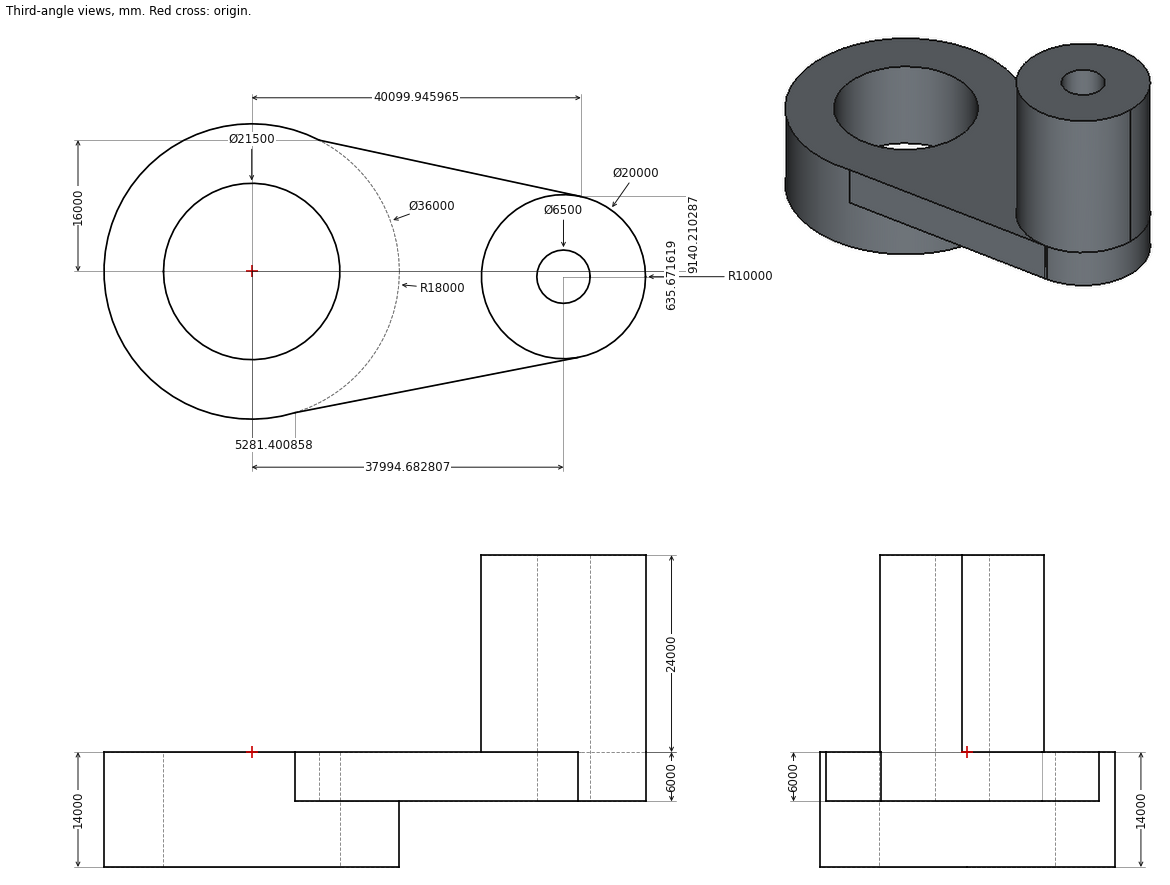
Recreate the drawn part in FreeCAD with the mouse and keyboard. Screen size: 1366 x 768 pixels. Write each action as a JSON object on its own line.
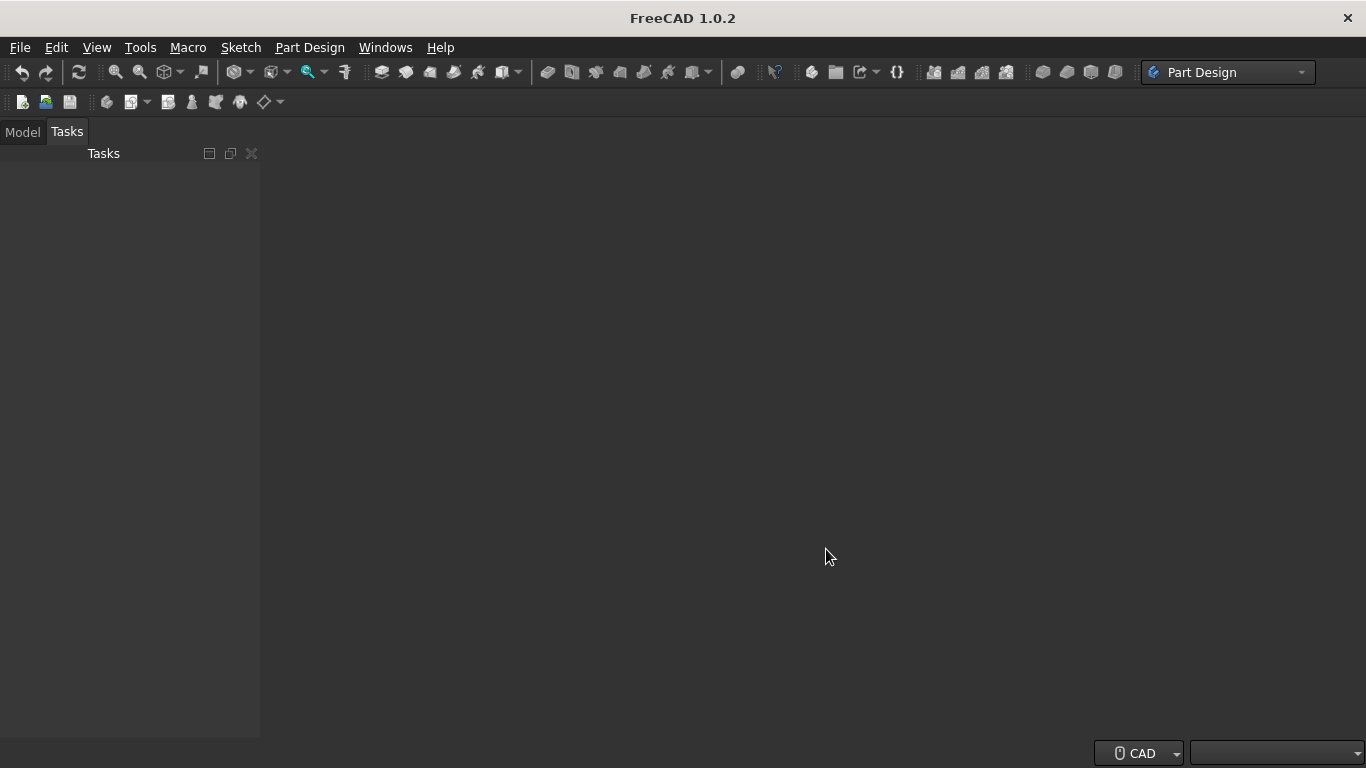
{"action": "left_click", "coordinate": [22, 102]}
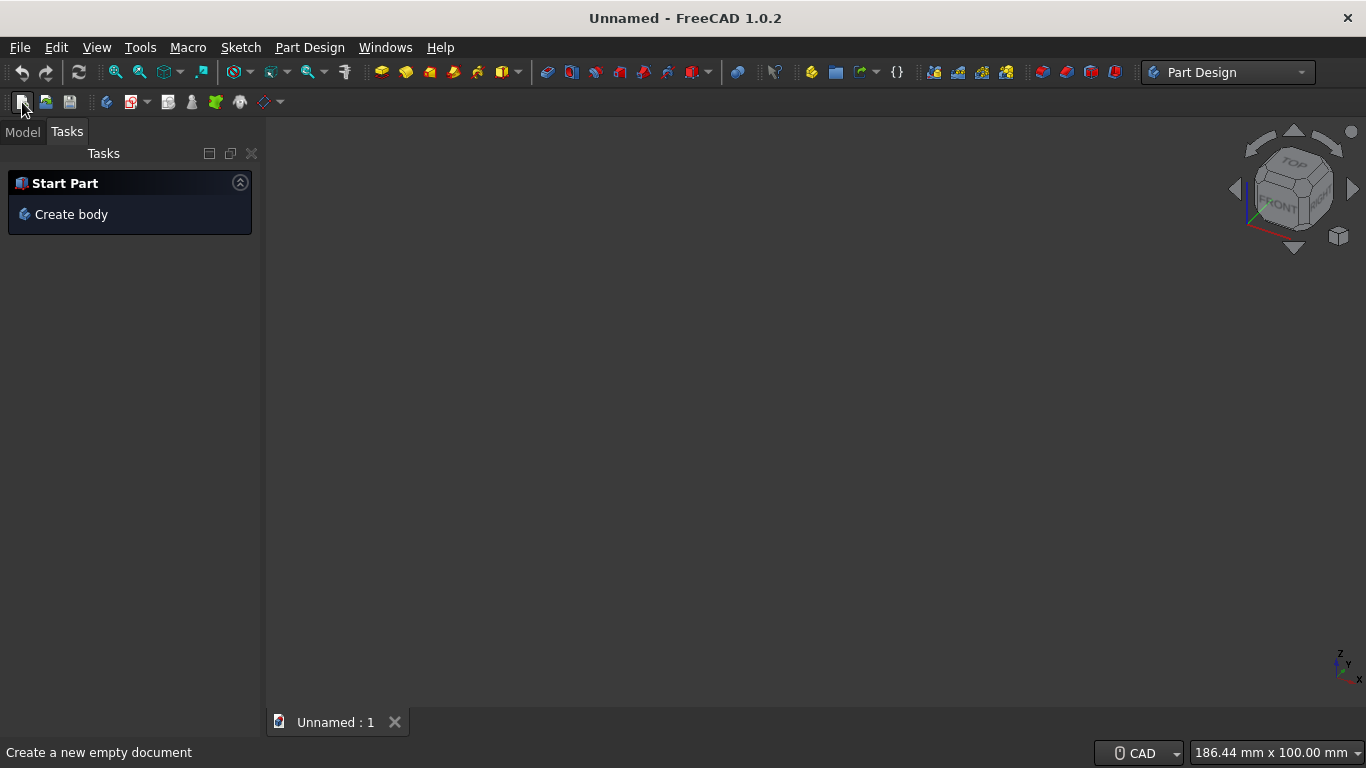
{"action": "left_click", "coordinate": [132, 102]}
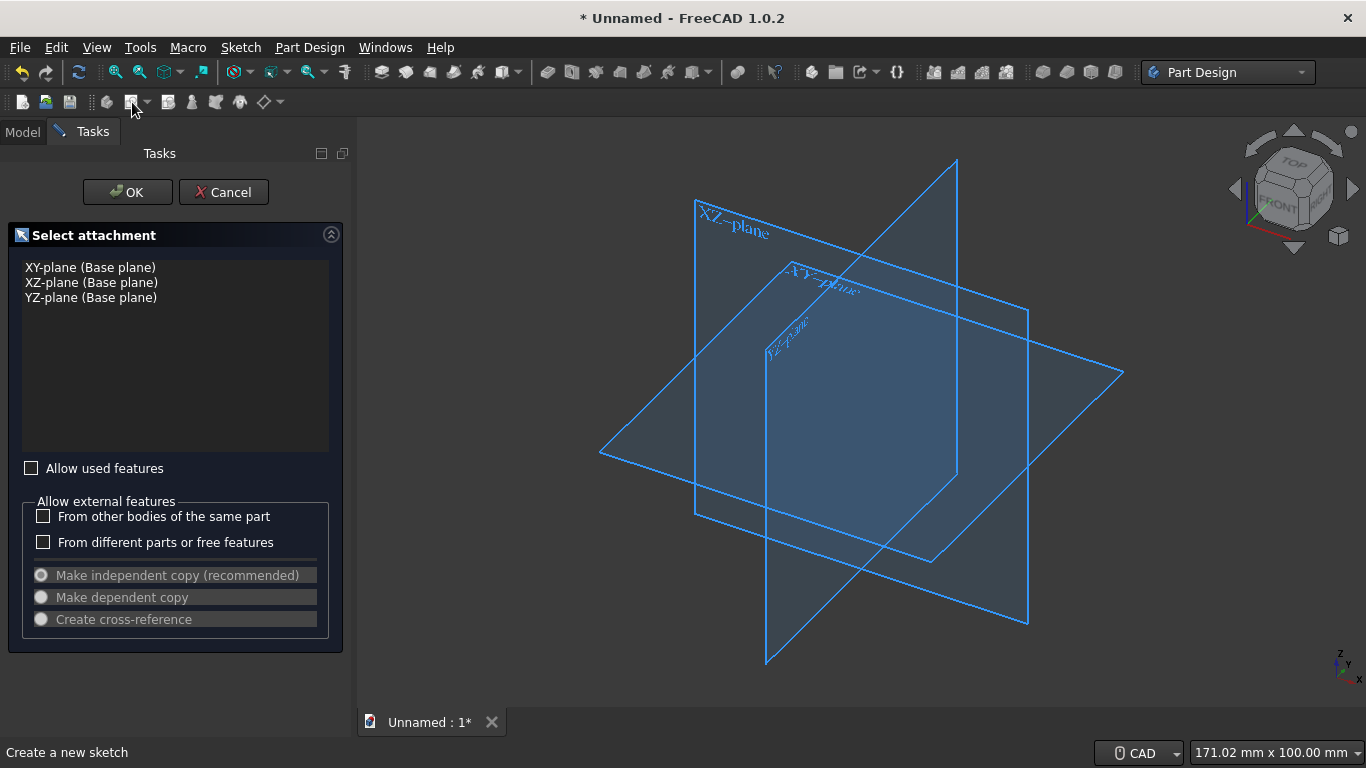
{"action": "left_click", "coordinate": [82, 268]}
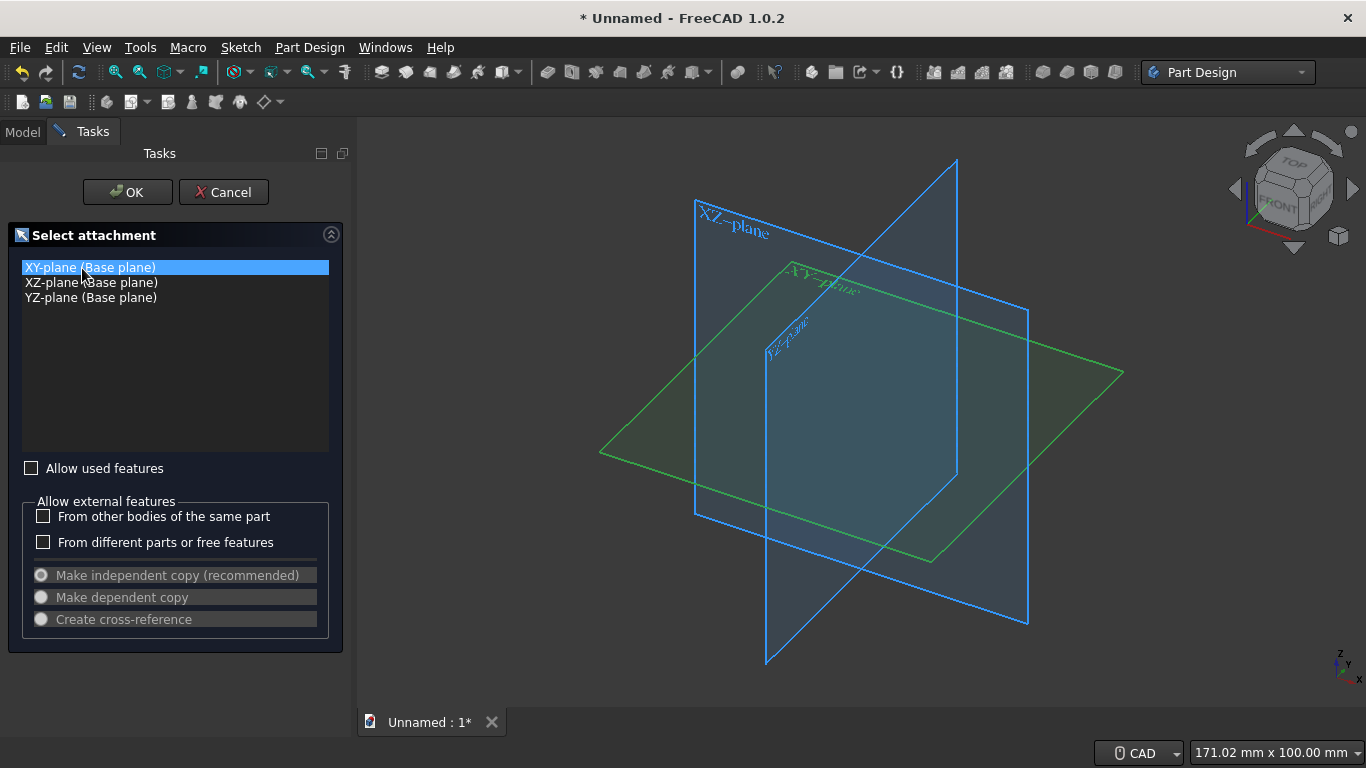
{"action": "left_click", "coordinate": [128, 192]}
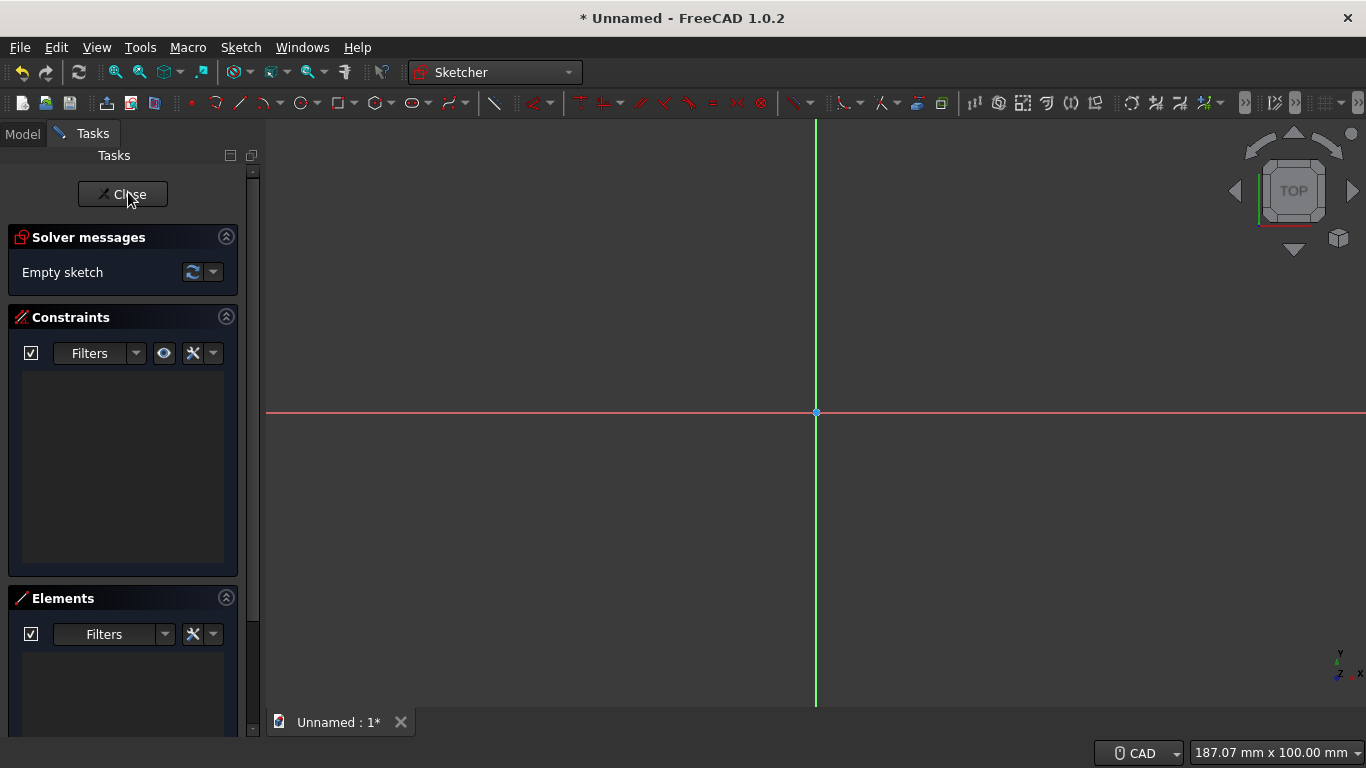
{"action": "scroll", "coordinate": [748, 413], "scroll_direction": "down", "scroll_amount": 15}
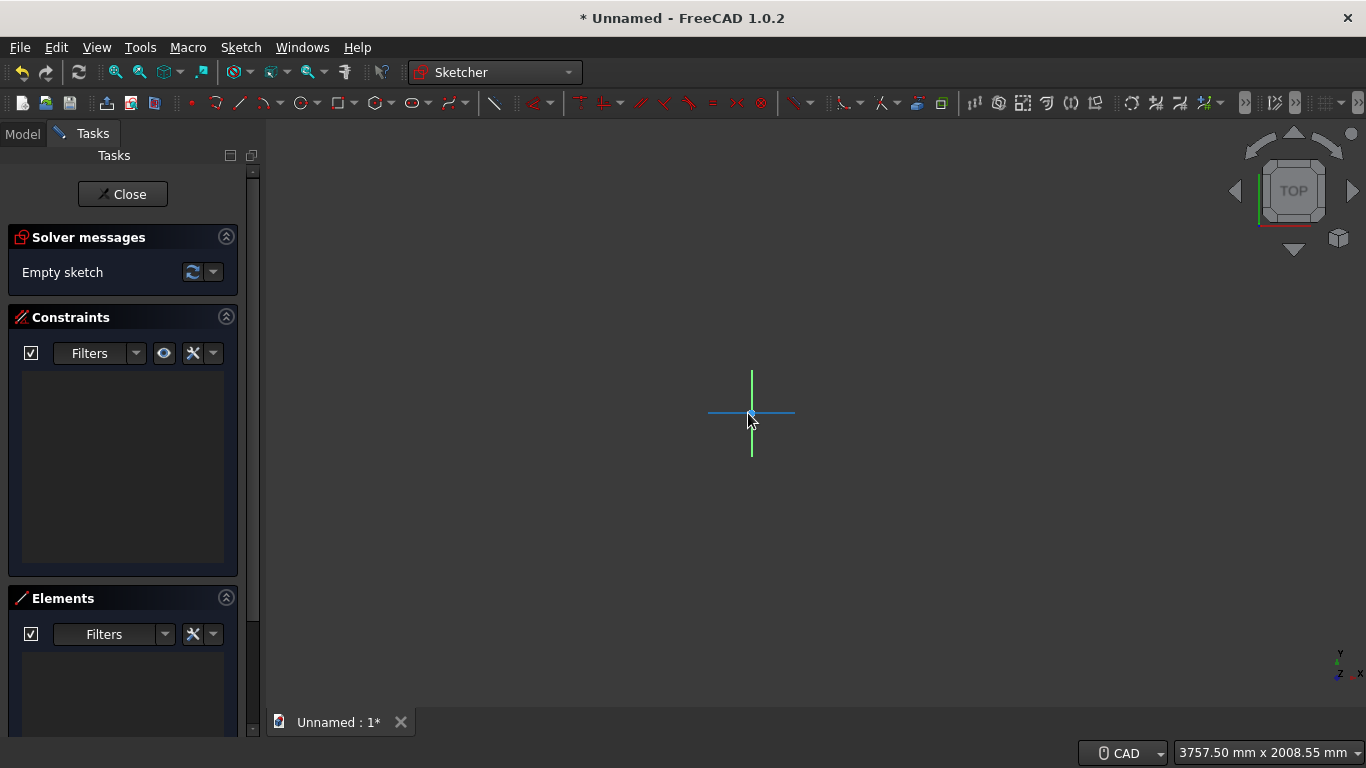
{"action": "scroll", "coordinate": [747, 413], "scroll_direction": "down", "scroll_amount": 16}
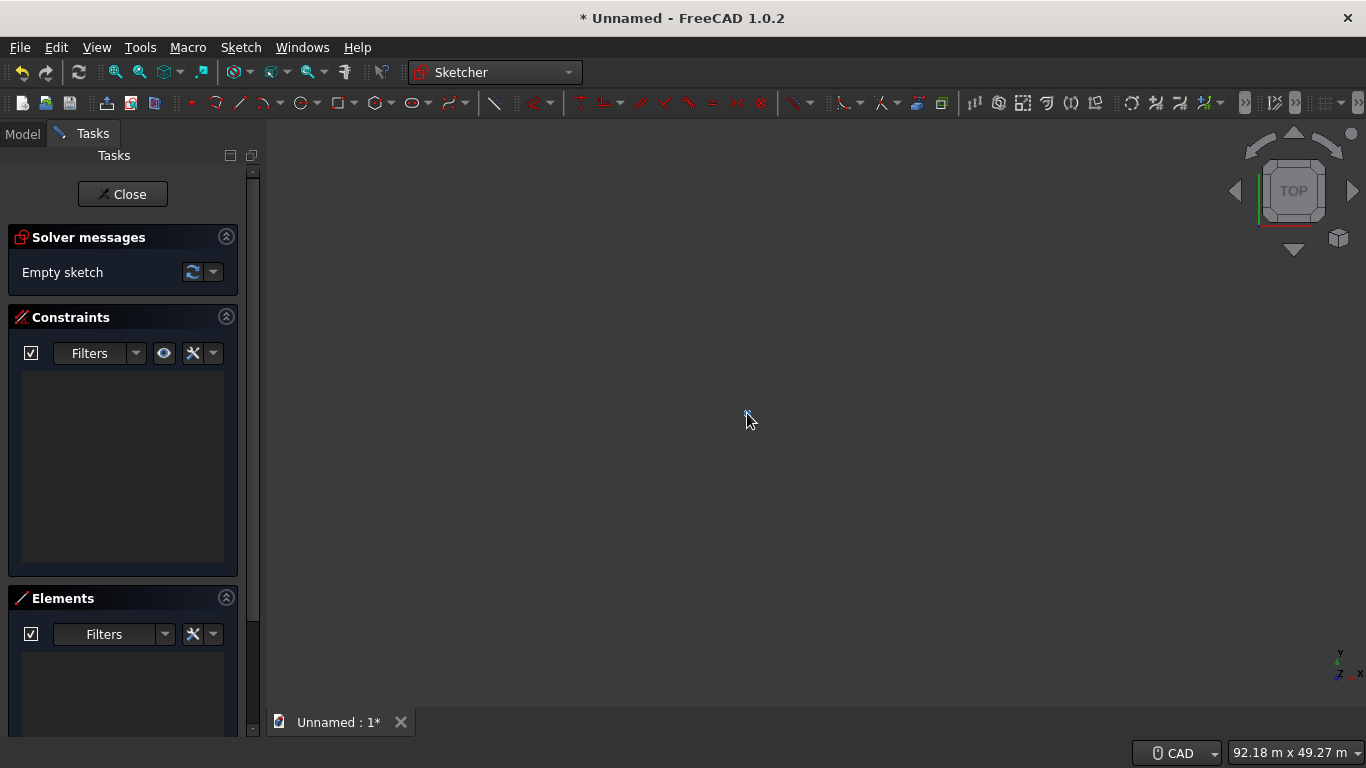
{"action": "left_click", "coordinate": [302, 104]}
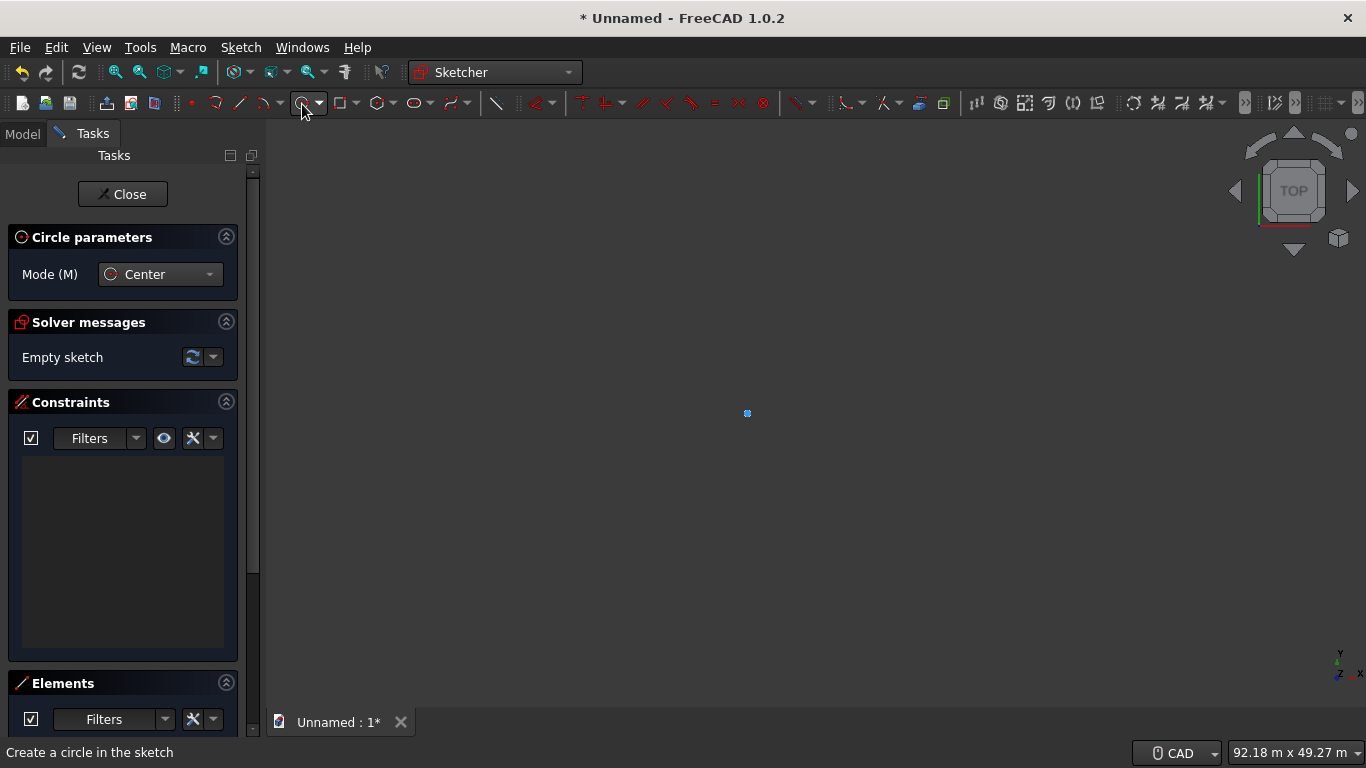
{"action": "left_click", "coordinate": [748, 413]}
{"action": "left_click", "coordinate": [899, 262]}
{"action": "key", "text": "Escape"}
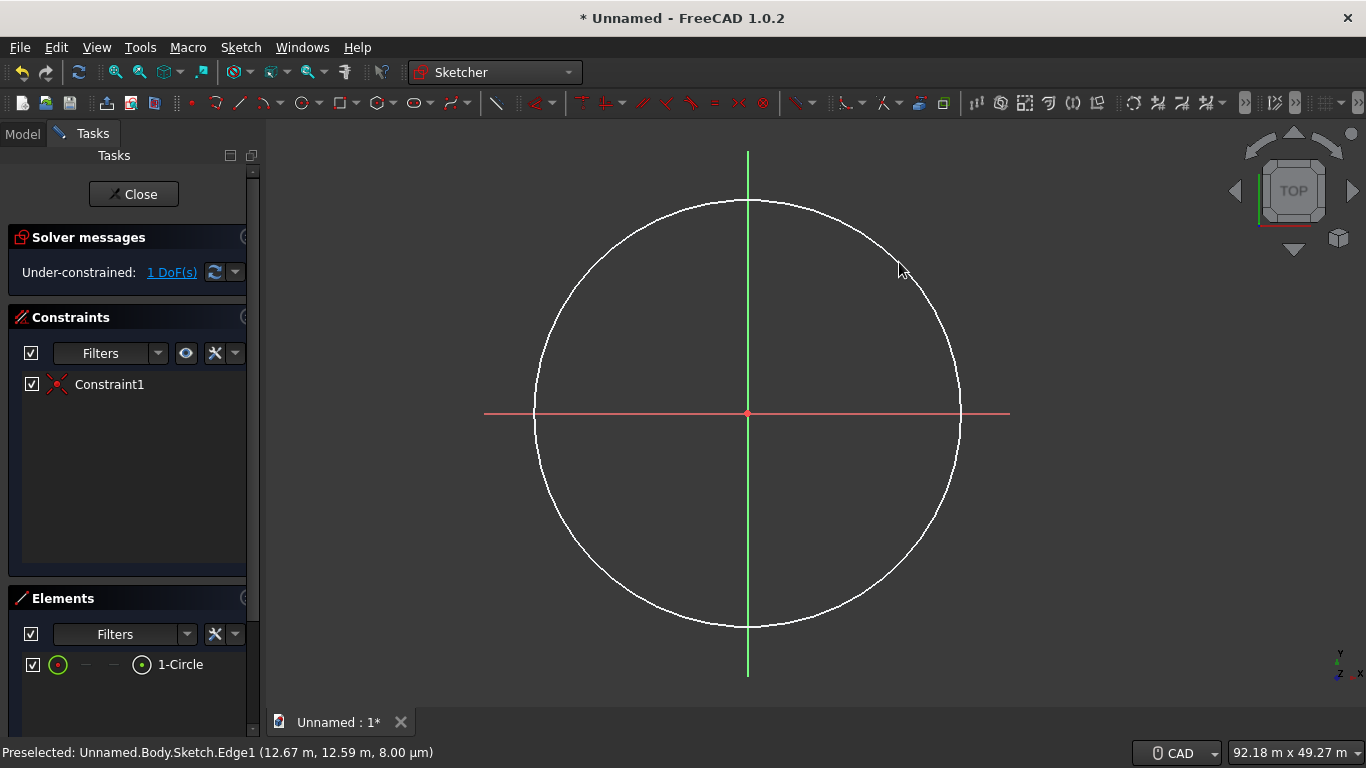
{"action": "left_click", "coordinate": [536, 104]}